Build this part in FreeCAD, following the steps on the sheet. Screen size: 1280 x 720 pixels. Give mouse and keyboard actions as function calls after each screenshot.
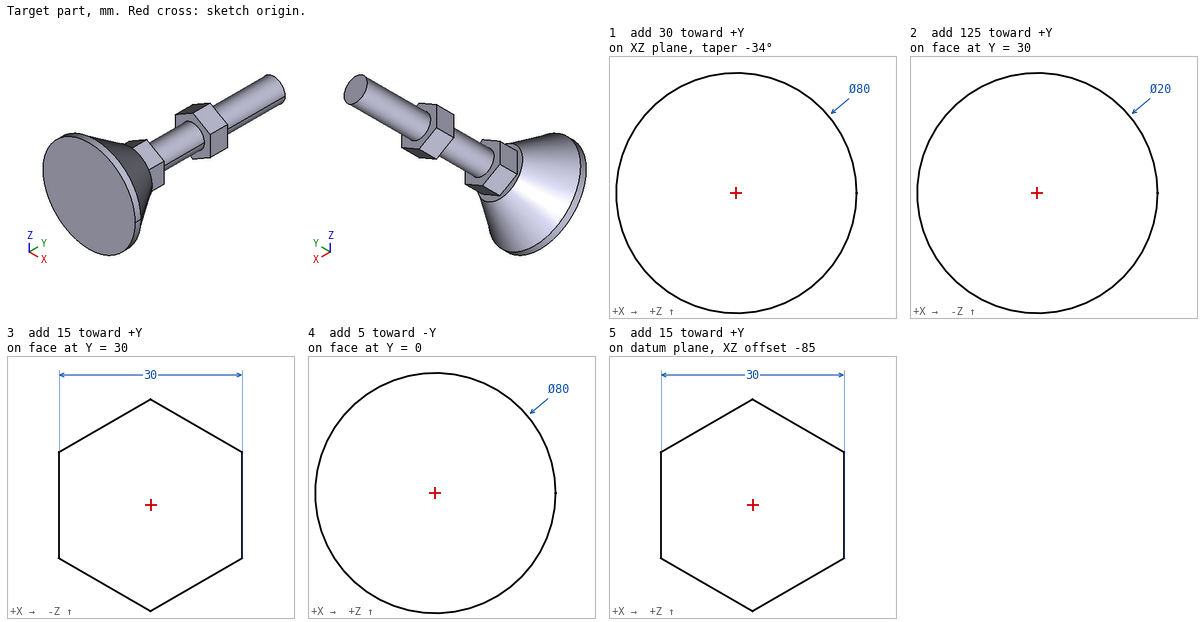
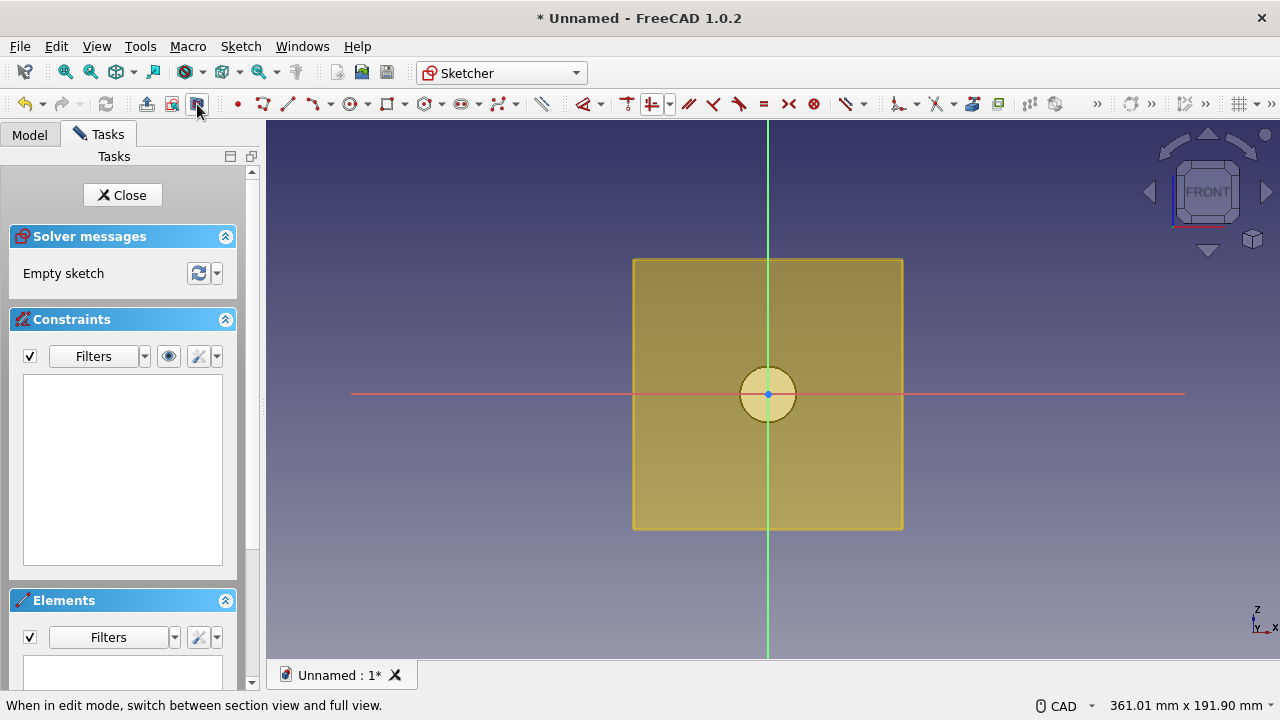
scroll(795, 397, up, 6)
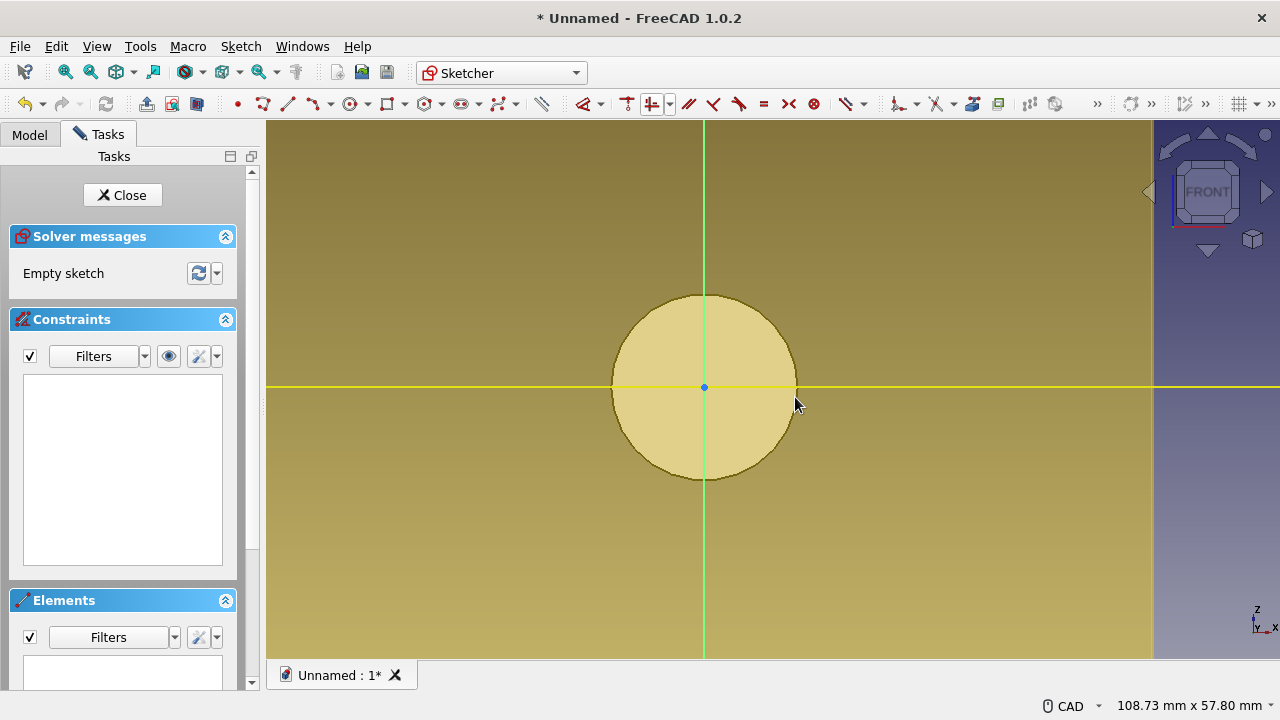
click(424, 104)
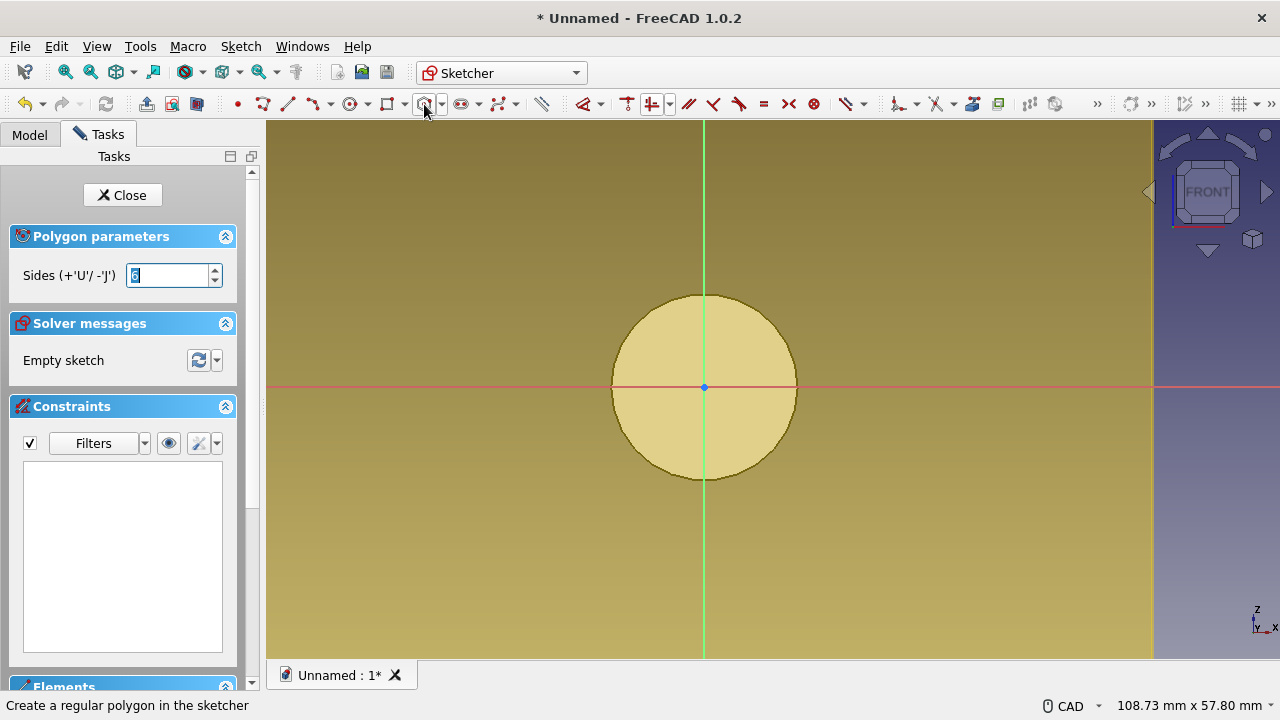
click(704, 387)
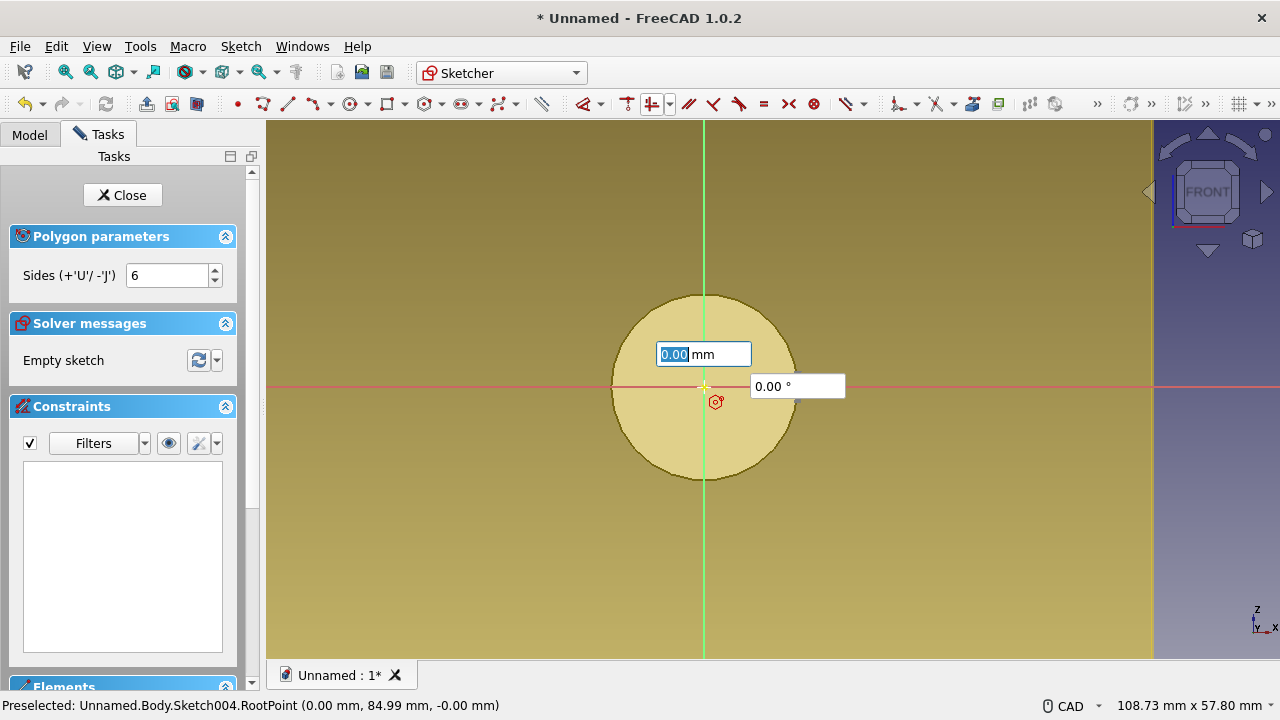
click(704, 226)
right_click(704, 226)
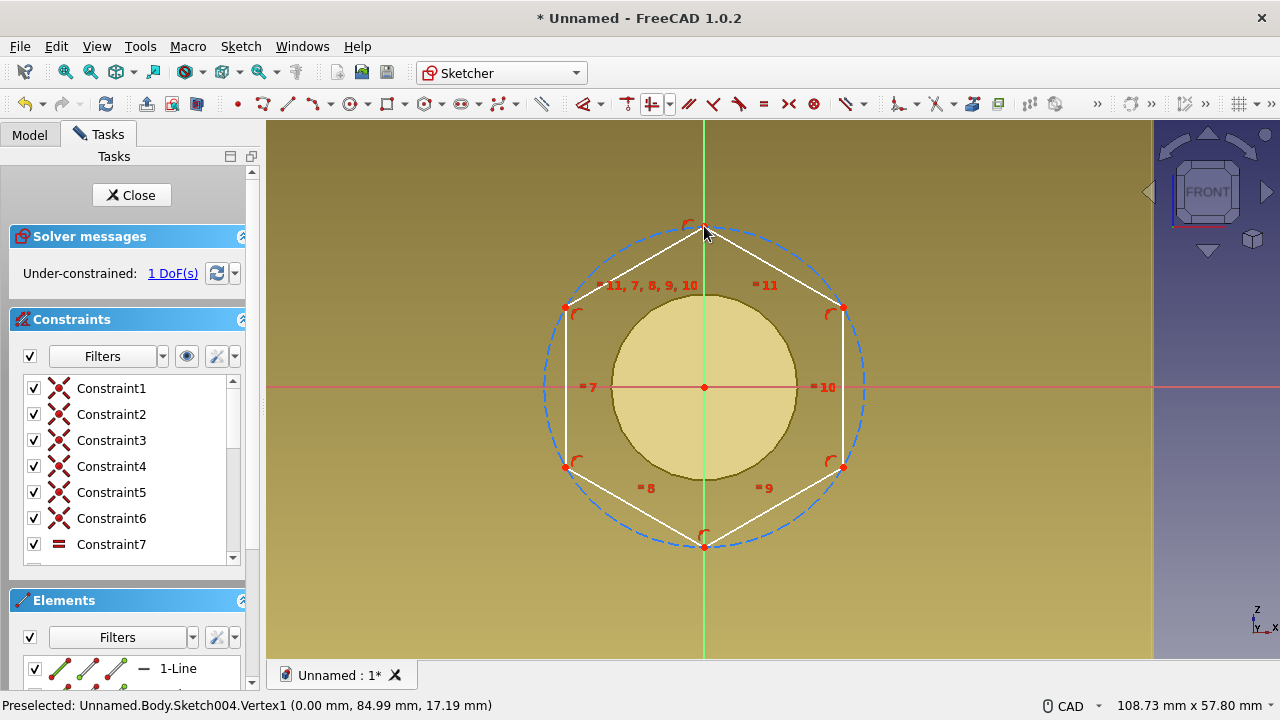
click(582, 104)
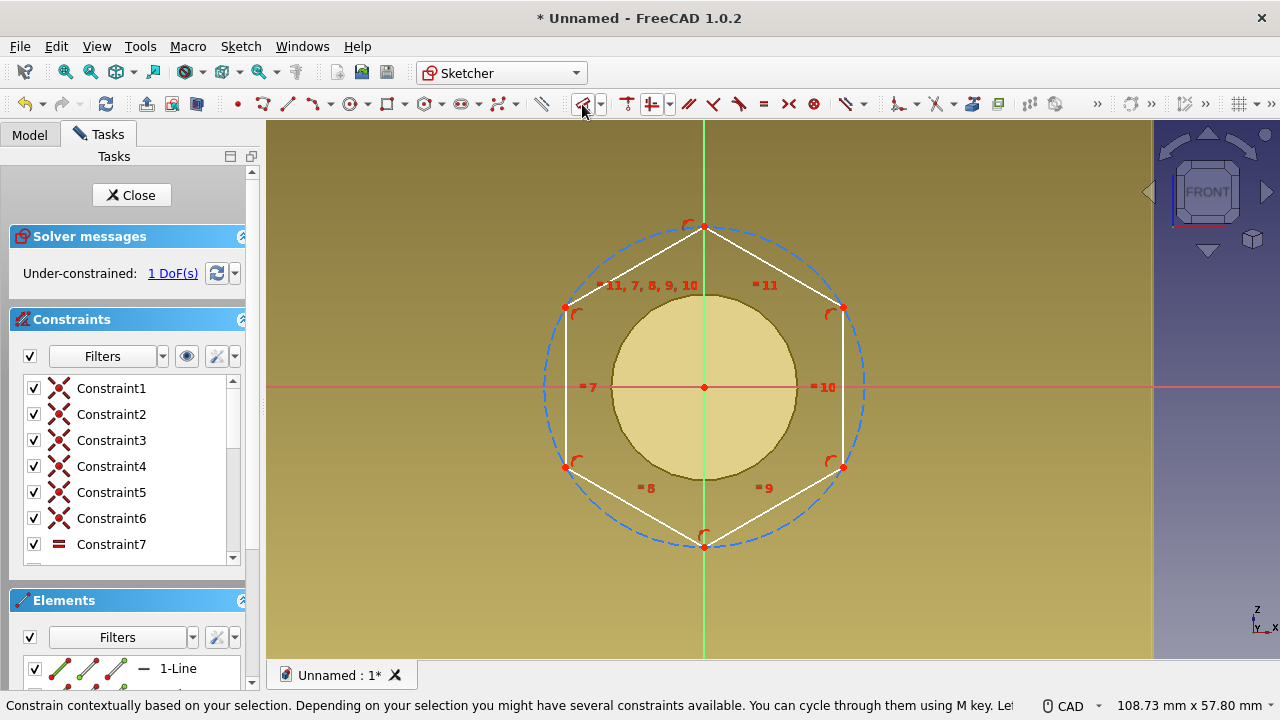
click(566, 307)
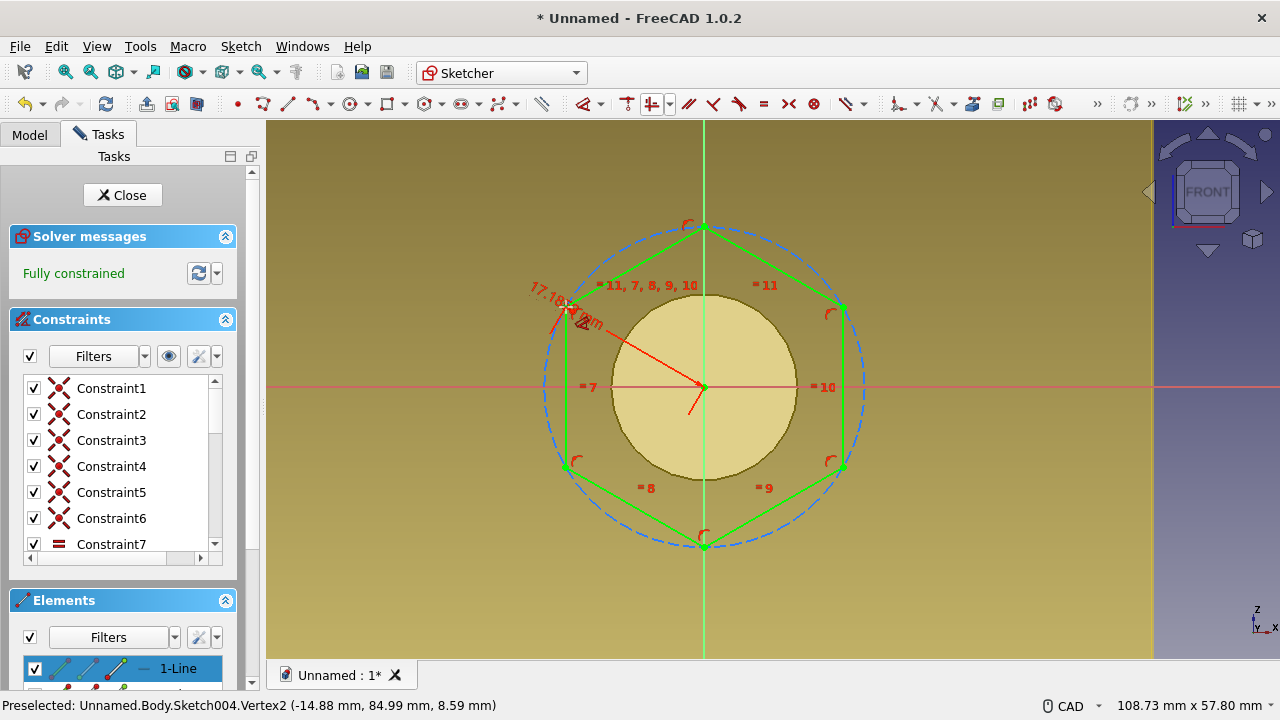
click(843, 467)
click(641, 549)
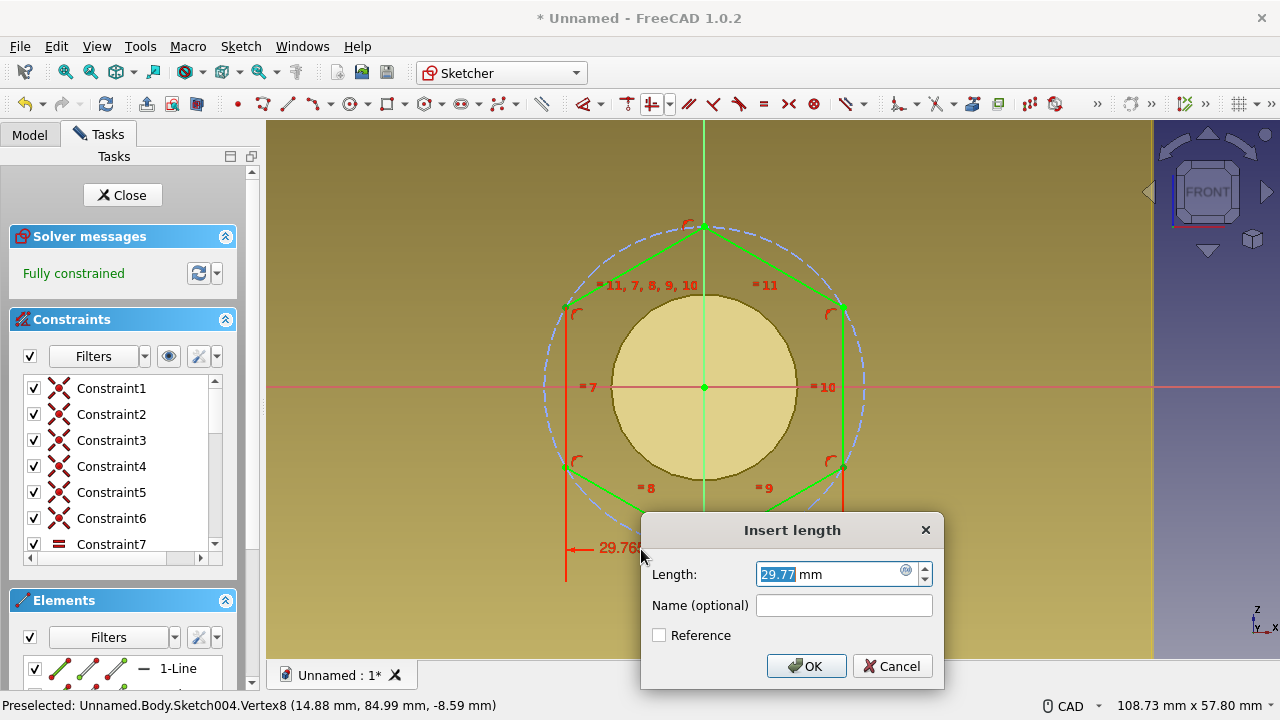
text(30)
key(Return)
key(Escape)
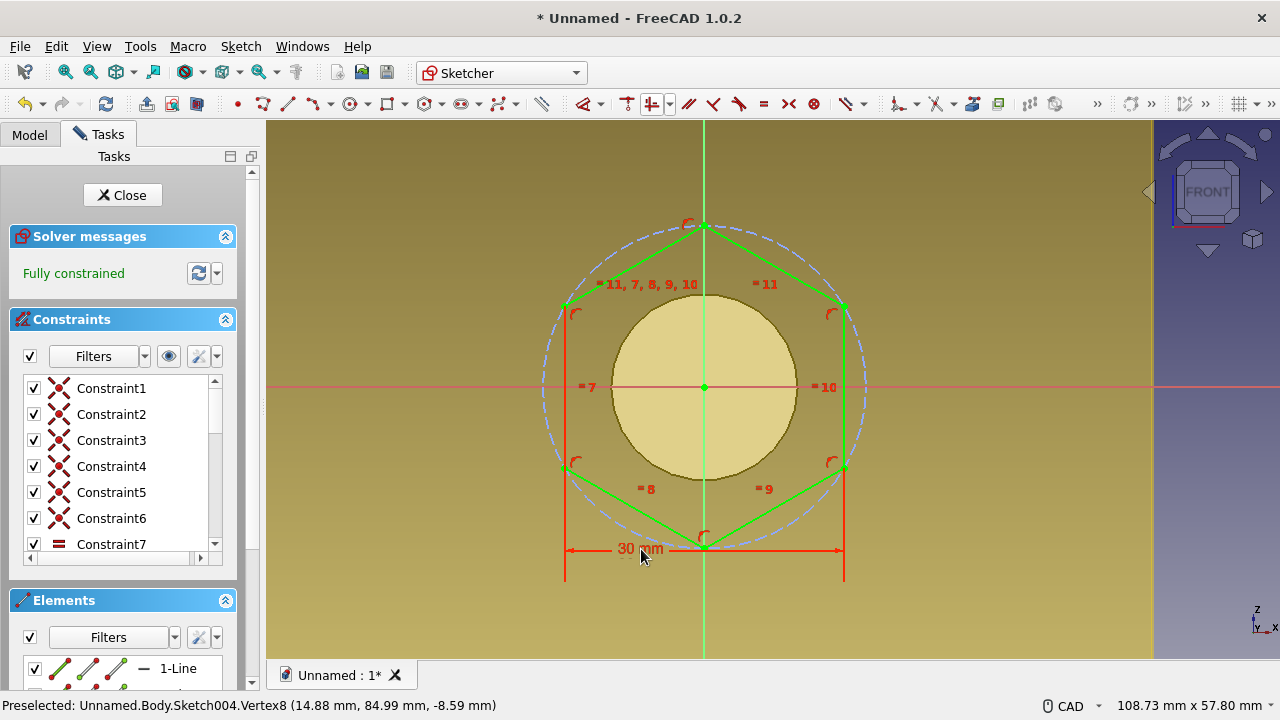
click(123, 195)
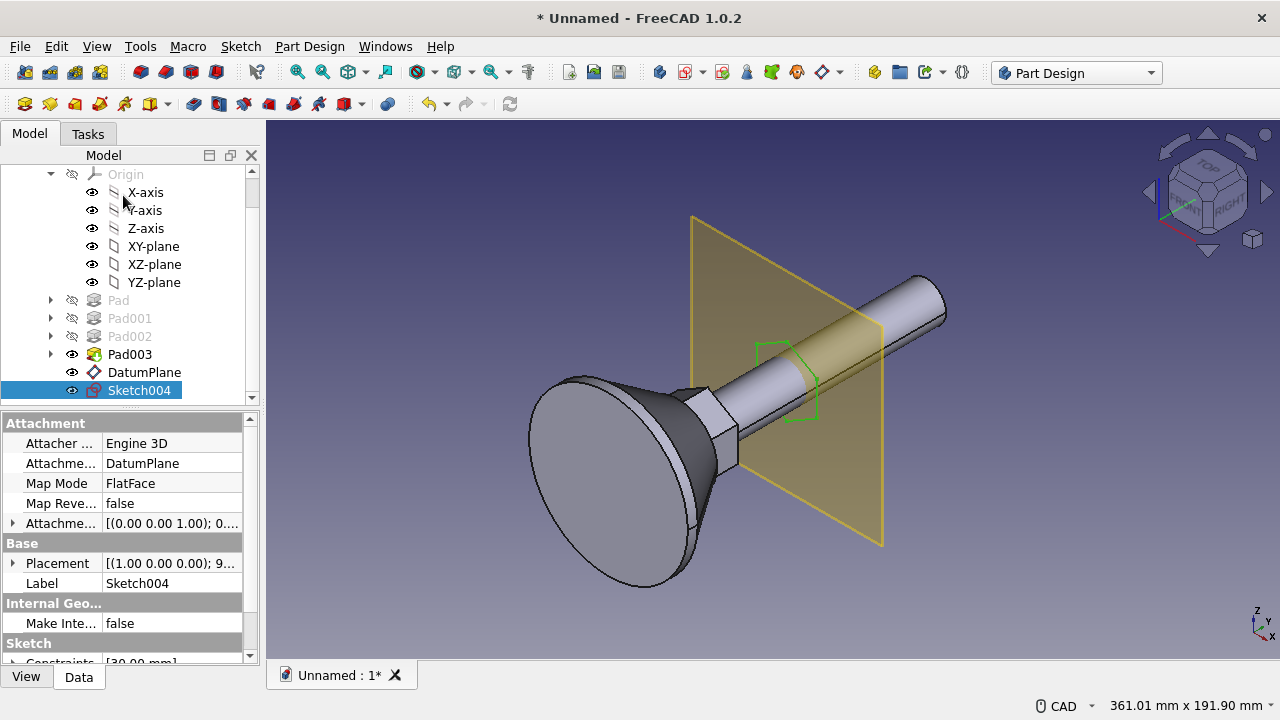
click(25, 104)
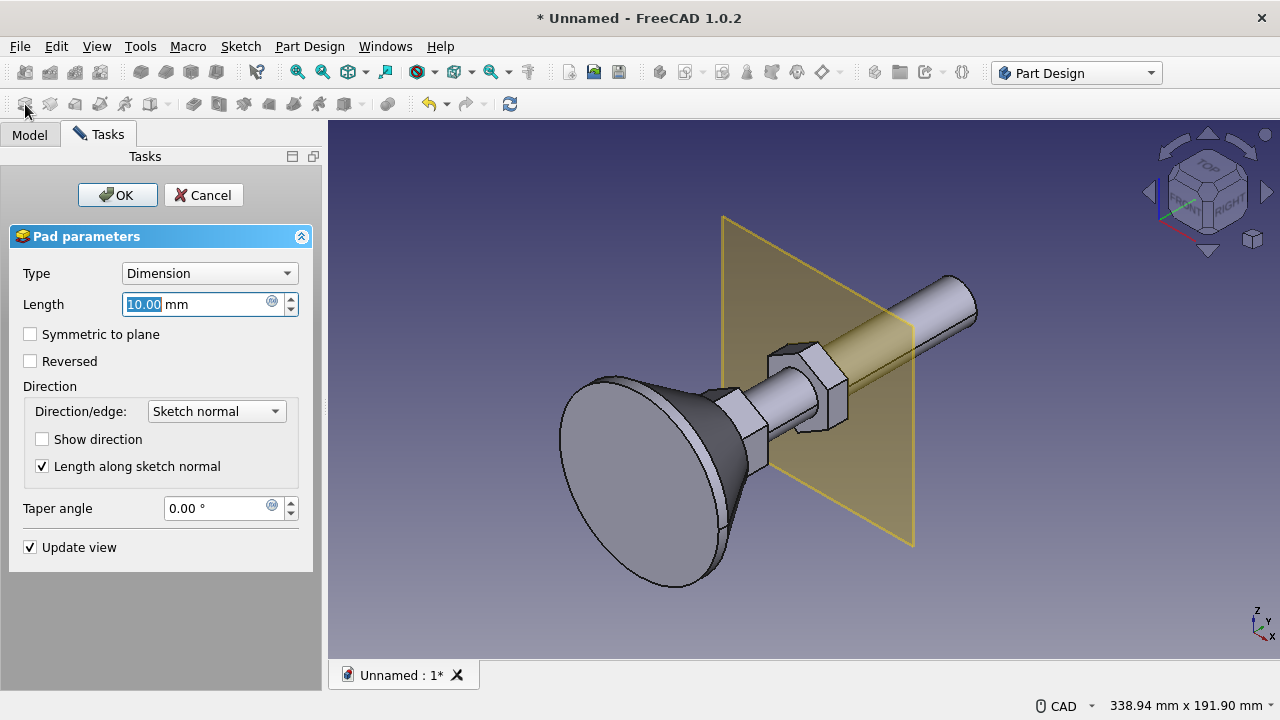
text(15)
key(Tab)